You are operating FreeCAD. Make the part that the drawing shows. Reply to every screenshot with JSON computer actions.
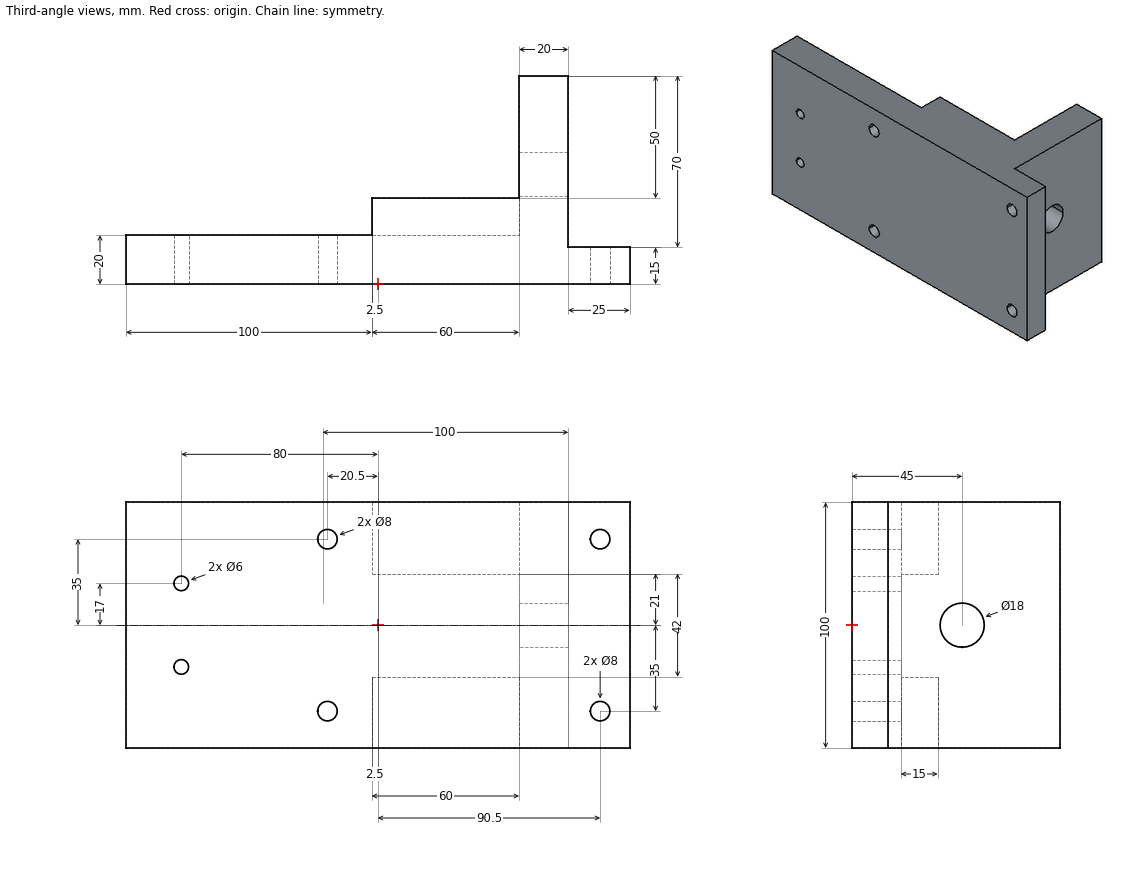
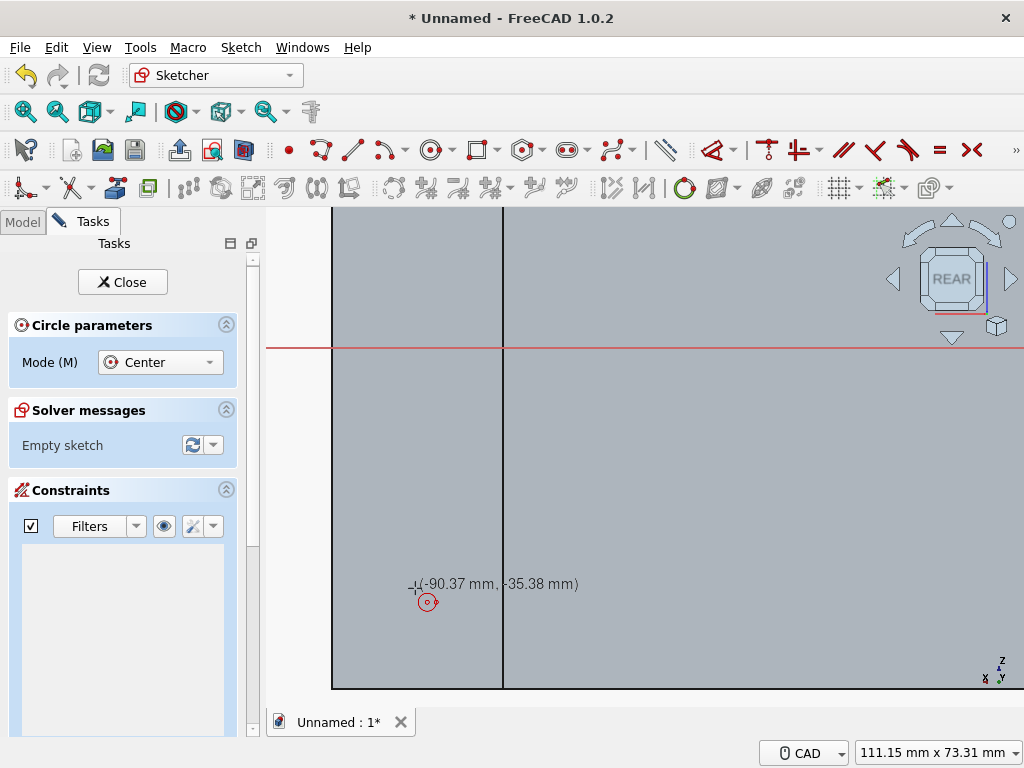
{"action": "left_click", "coordinate": [414, 587]}
{"action": "left_click", "coordinate": [433, 567]}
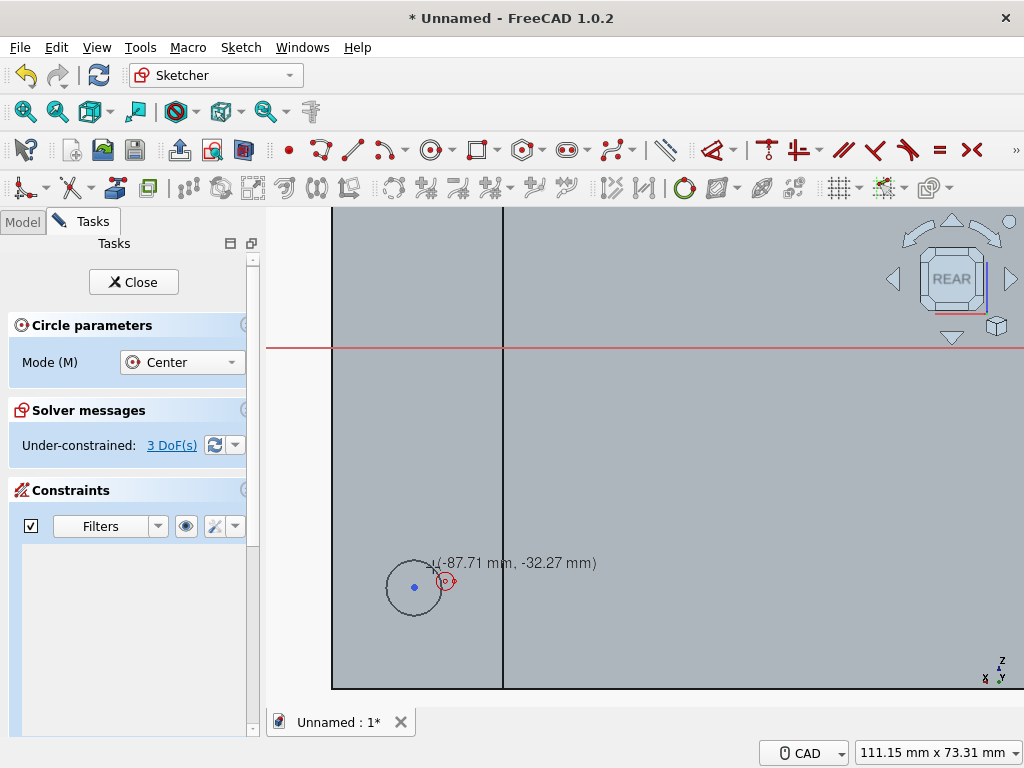
{"action": "scroll", "coordinate": [415, 590], "scroll_direction": "down", "scroll_amount": 3}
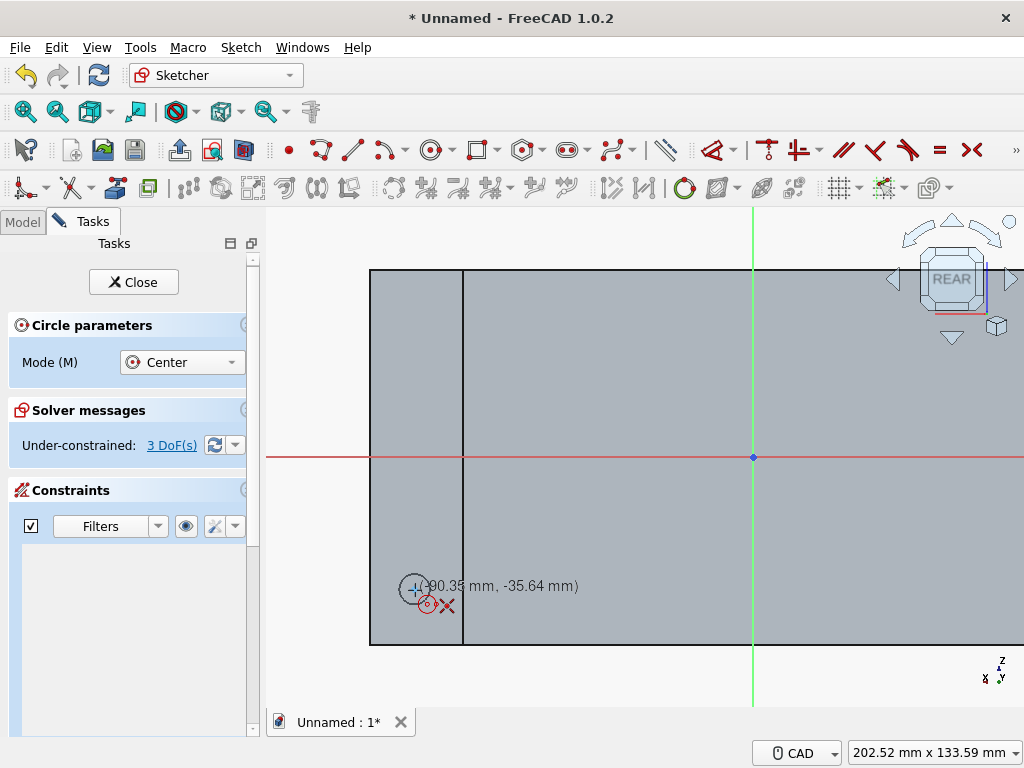
{"action": "scroll", "coordinate": [415, 326], "scroll_direction": "up", "scroll_amount": 3}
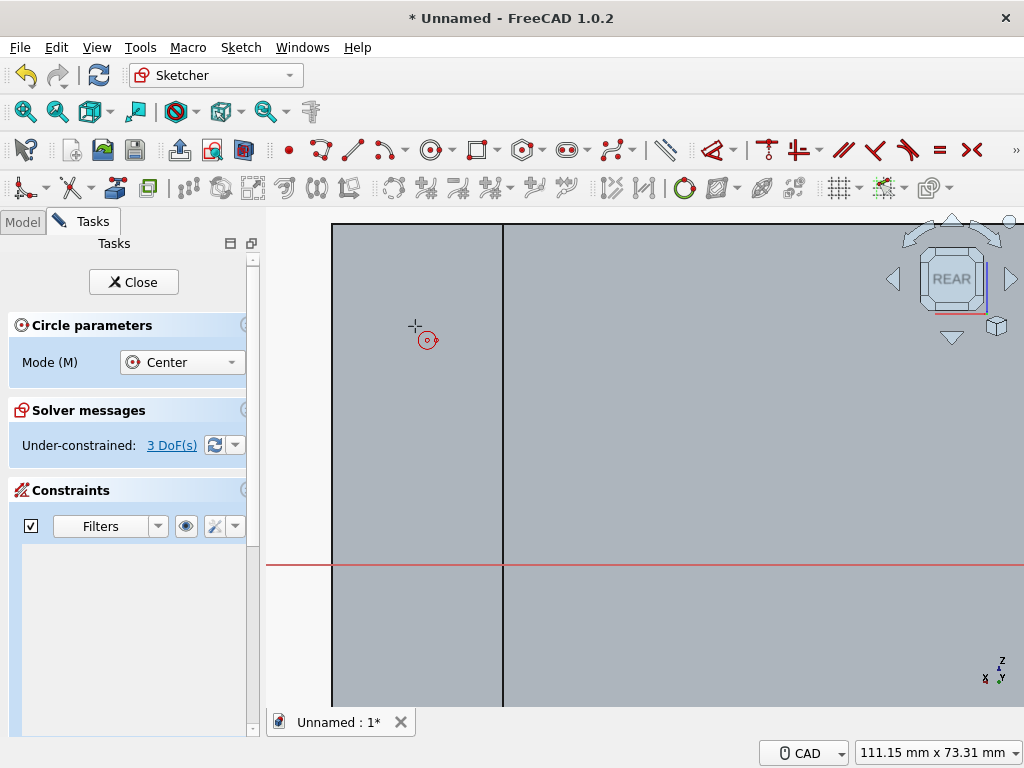
{"action": "left_click", "coordinate": [414, 327]}
{"action": "left_click", "coordinate": [433, 307]}
{"action": "key", "text": "Escape"}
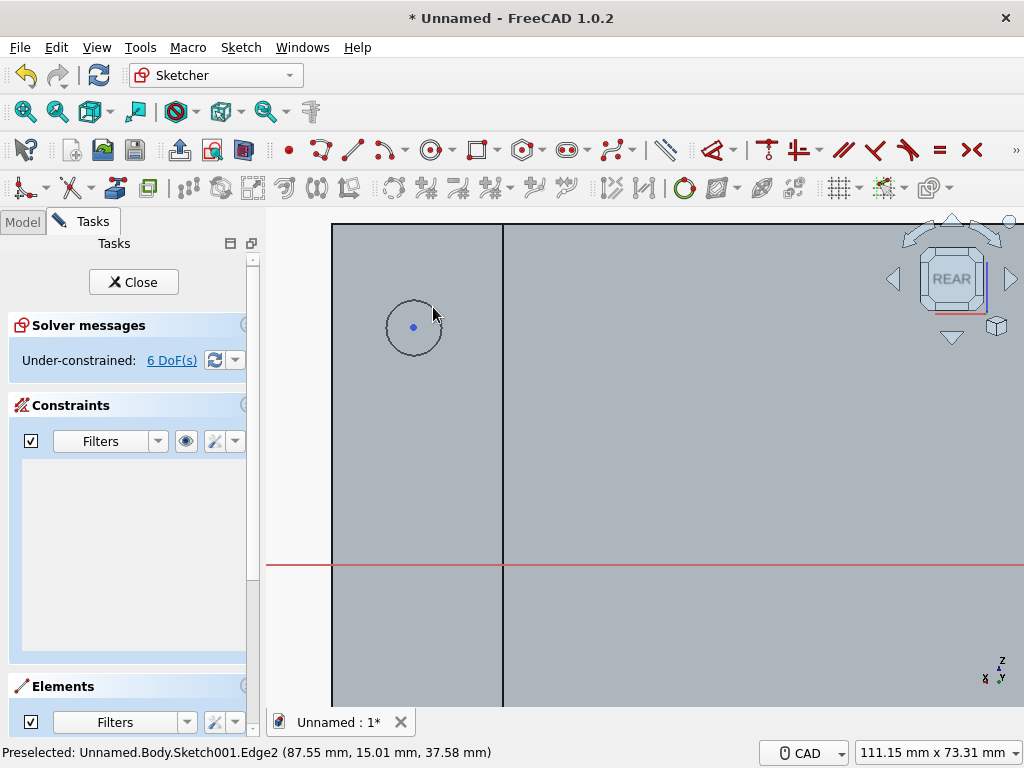
{"action": "scroll", "coordinate": [415, 325], "scroll_direction": "down", "scroll_amount": 3}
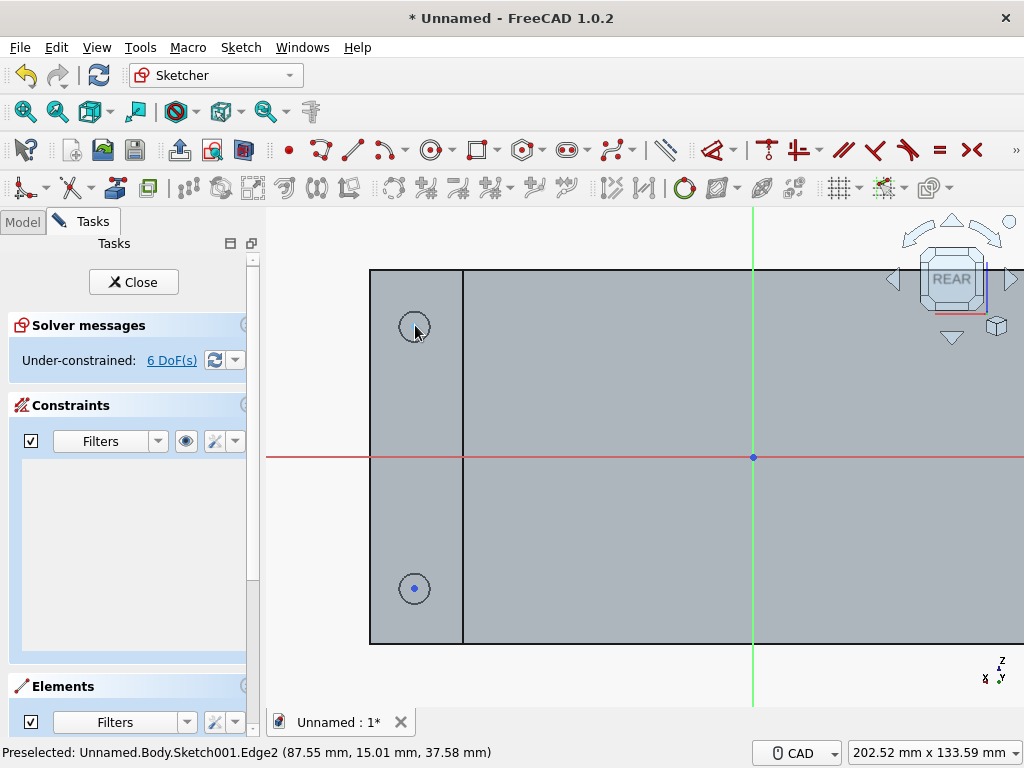
{"action": "left_click", "coordinate": [425, 578]}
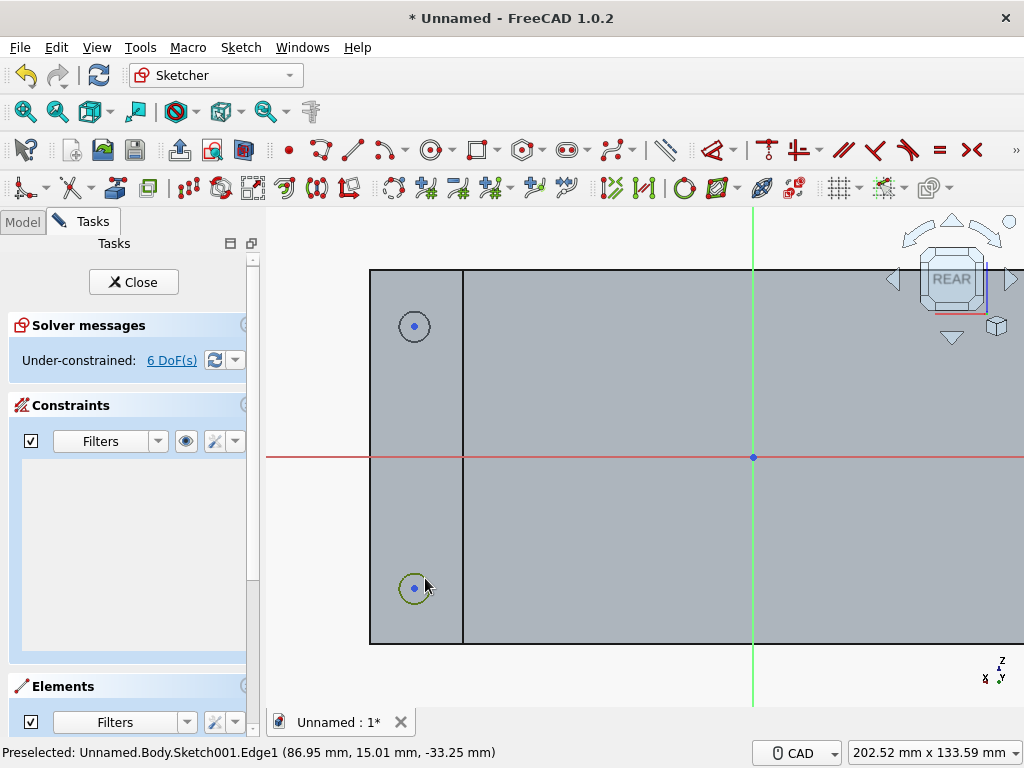
{"action": "left_click", "coordinate": [425, 316]}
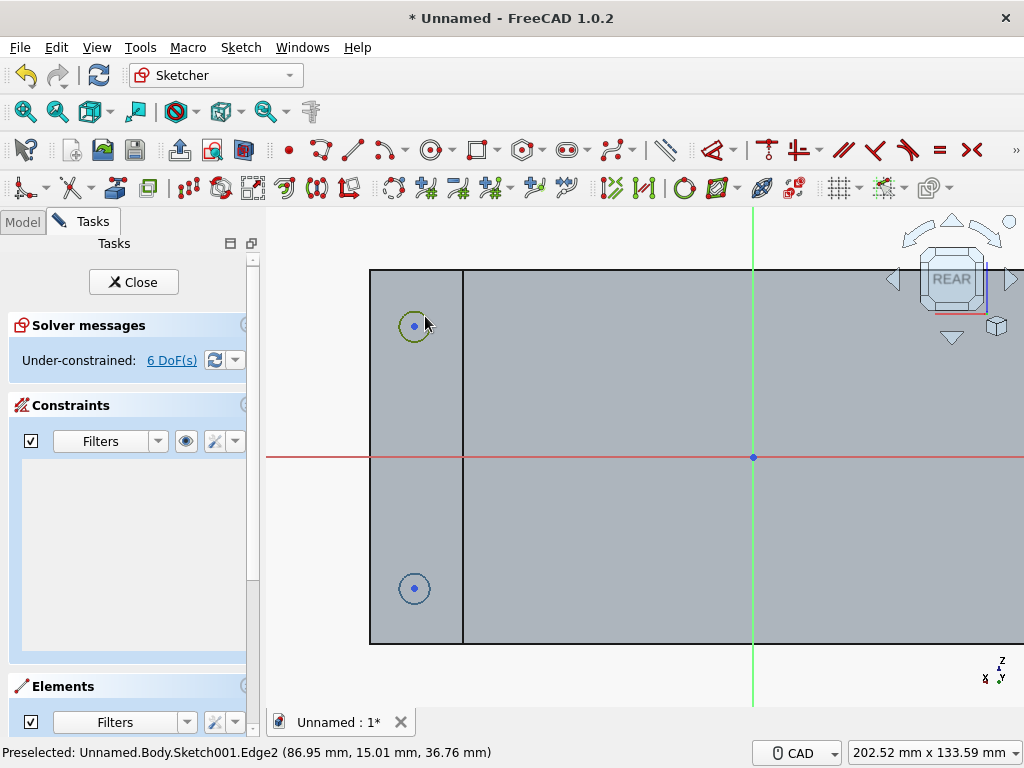
{"action": "left_click", "coordinate": [940, 150]}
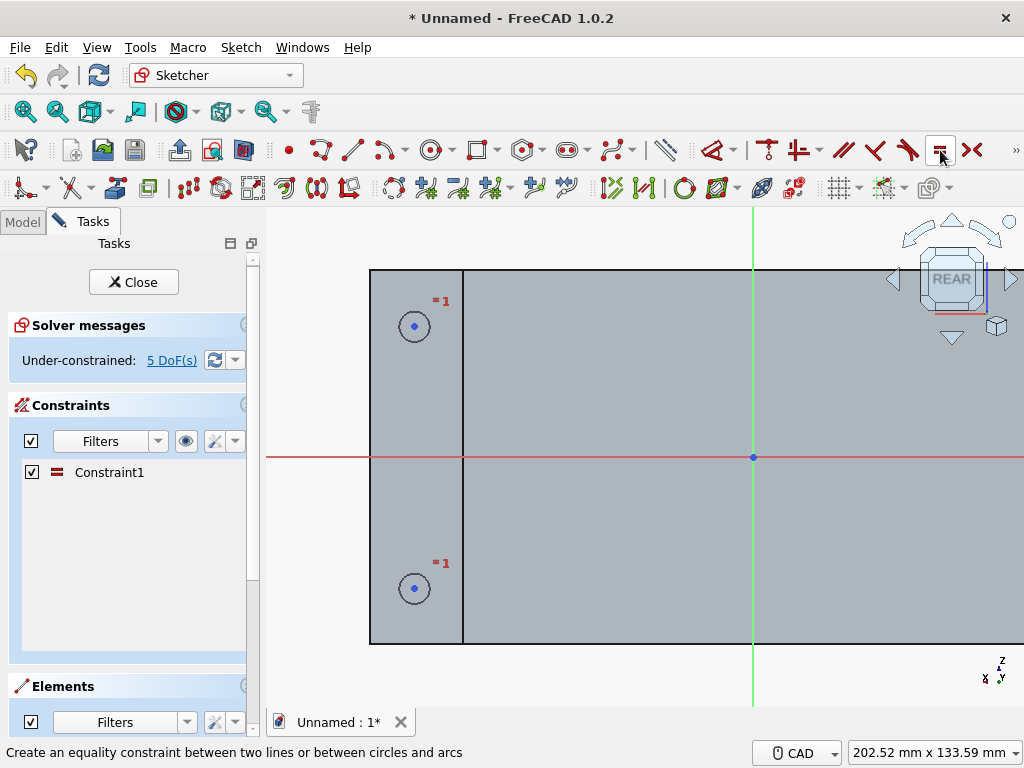
{"action": "left_click", "coordinate": [415, 589]}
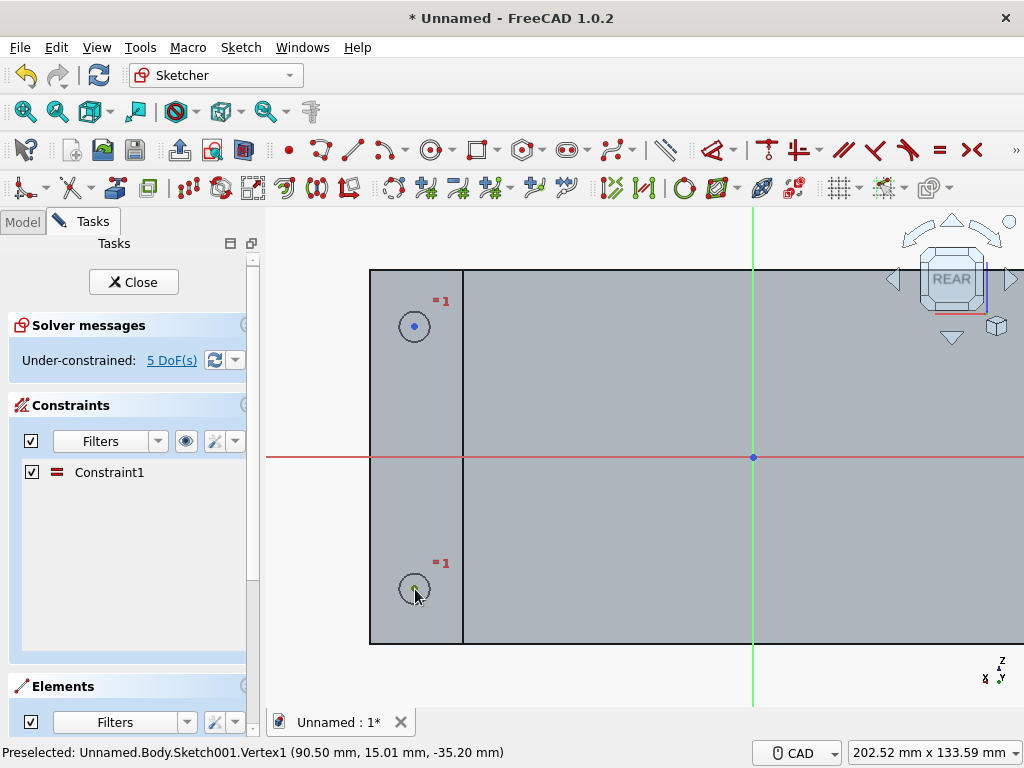
{"action": "left_click", "coordinate": [415, 327]}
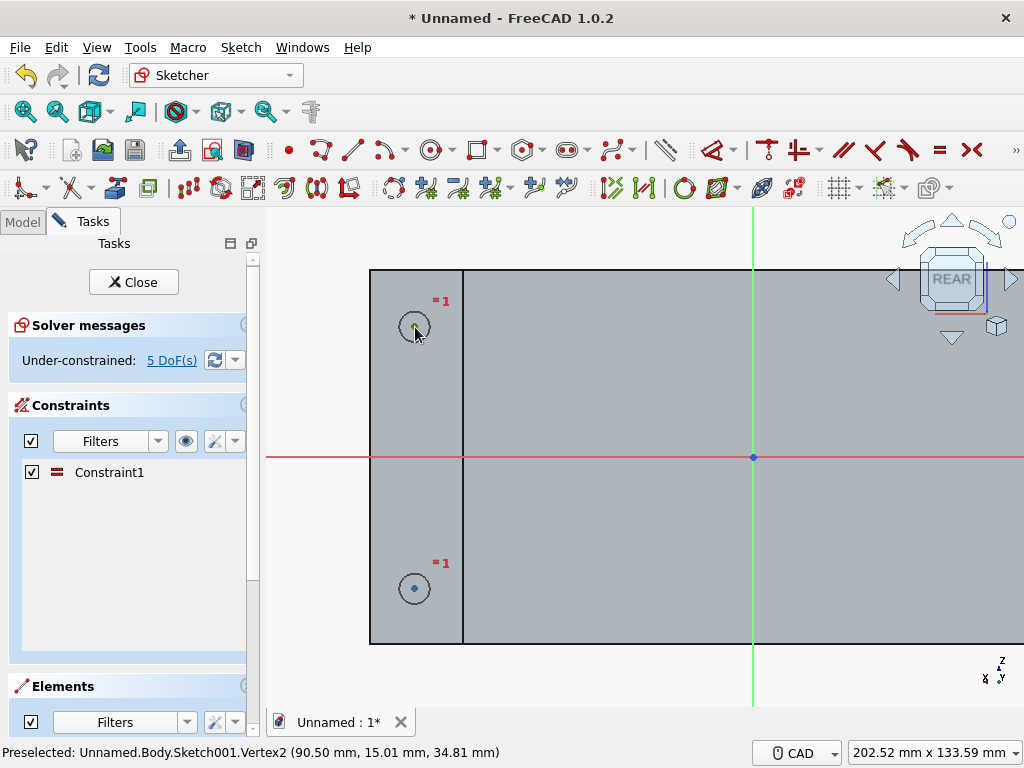
{"action": "left_click", "coordinate": [334, 457]}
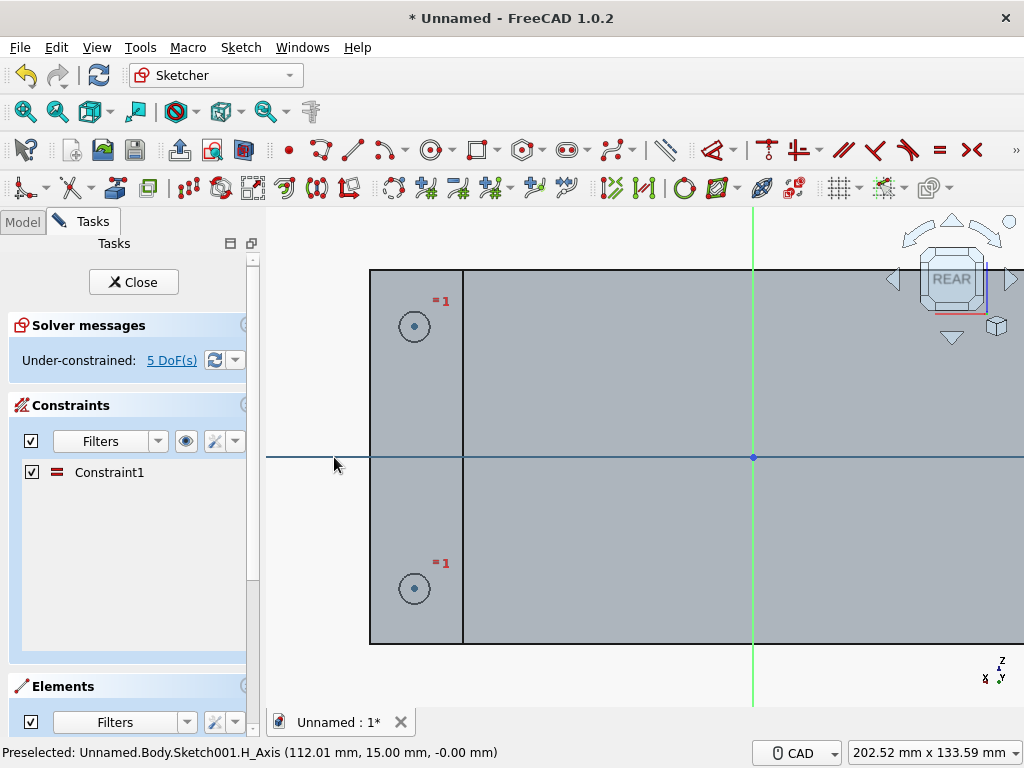
{"action": "left_click", "coordinate": [972, 150]}